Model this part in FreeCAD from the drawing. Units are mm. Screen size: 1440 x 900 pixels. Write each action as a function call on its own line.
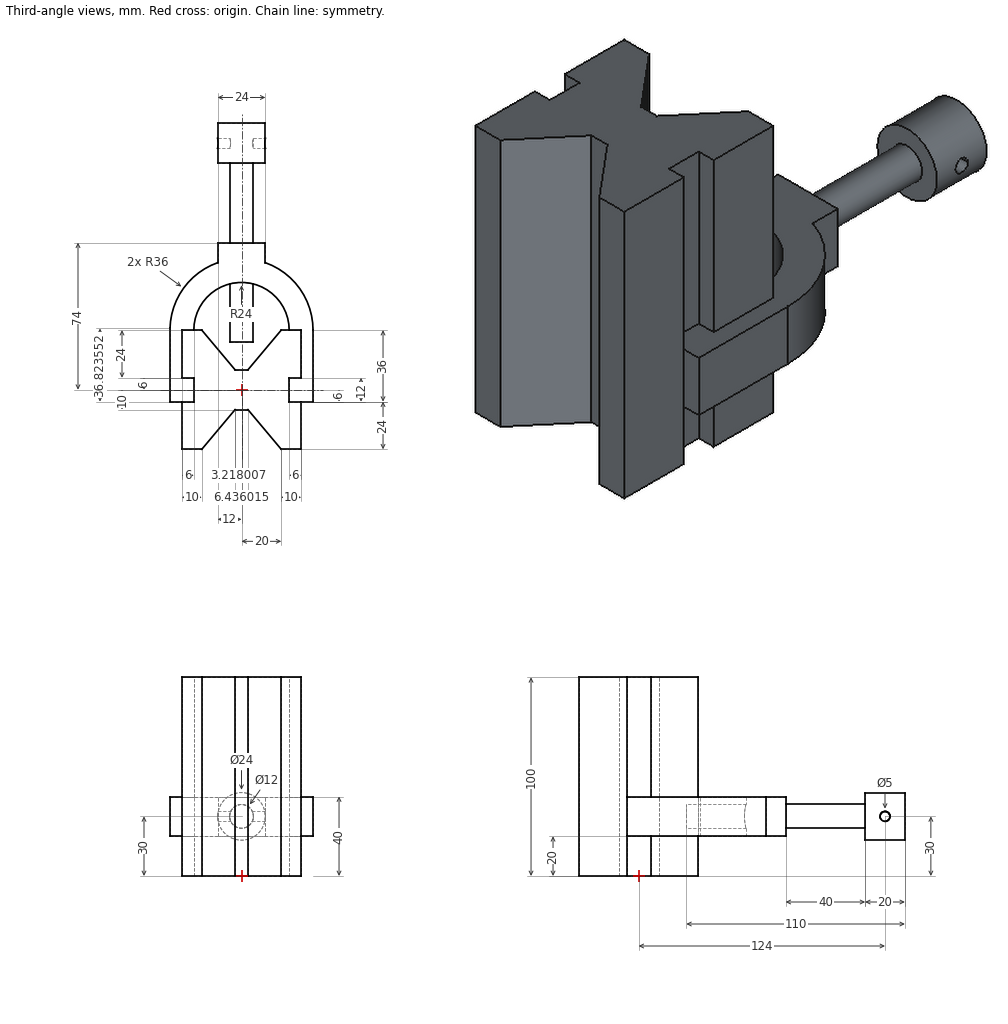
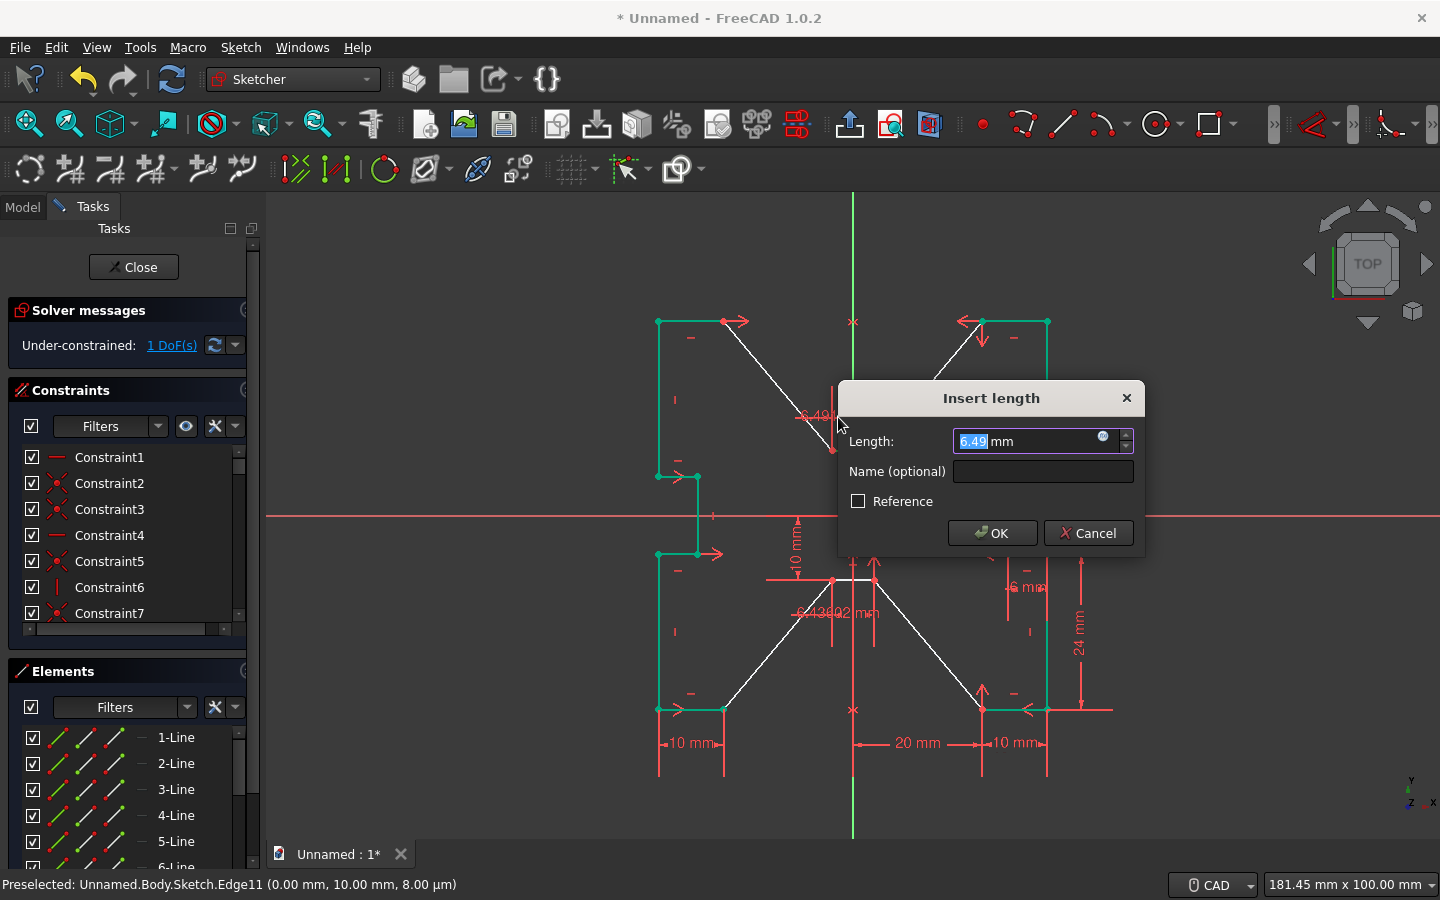
text(6.436015)
key(Return)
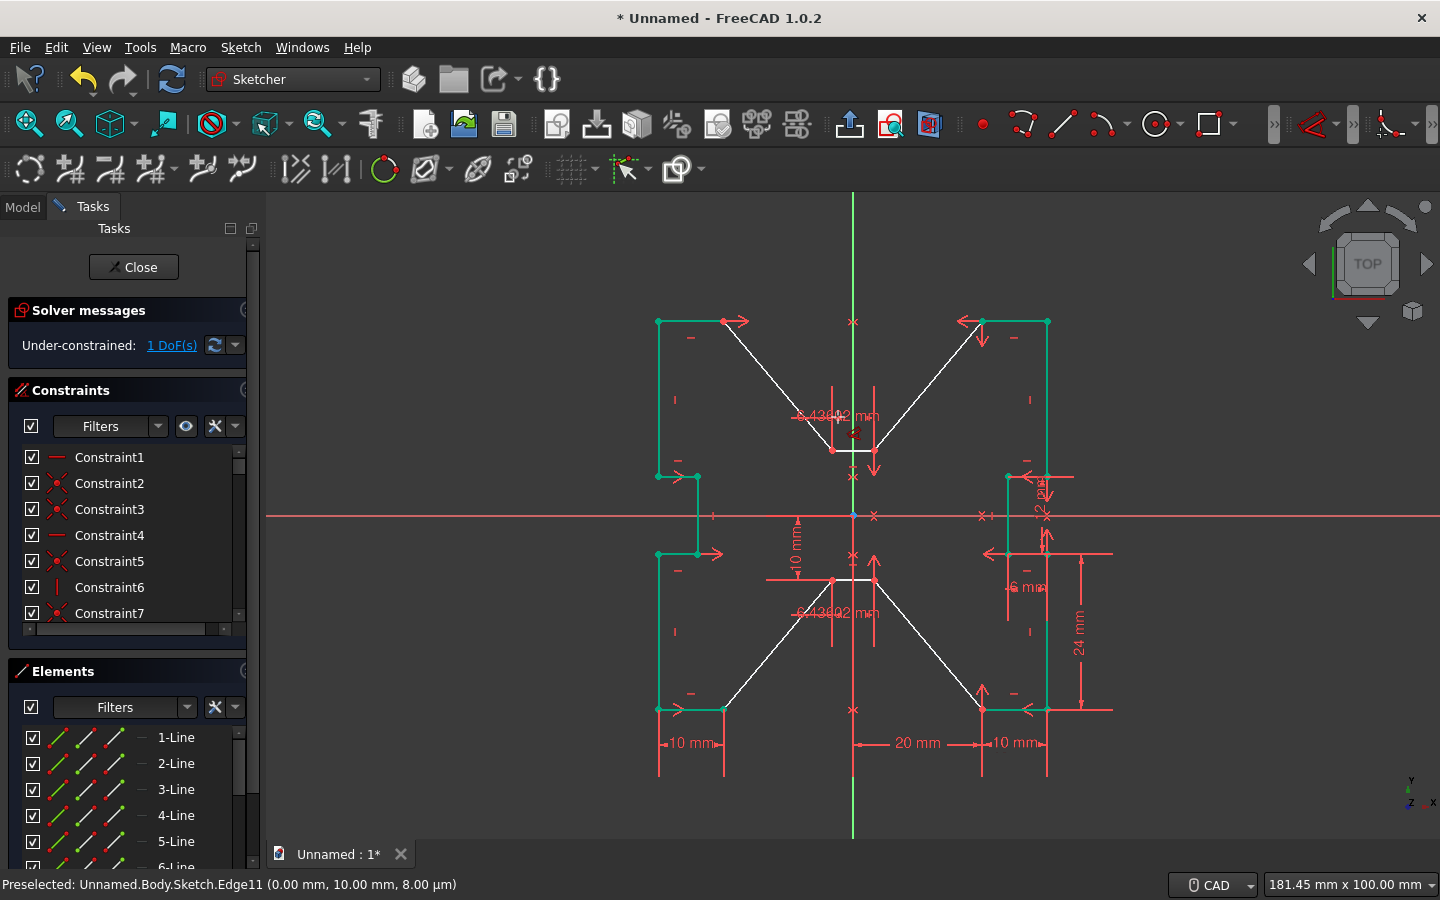
scroll(832, 580, up, 4)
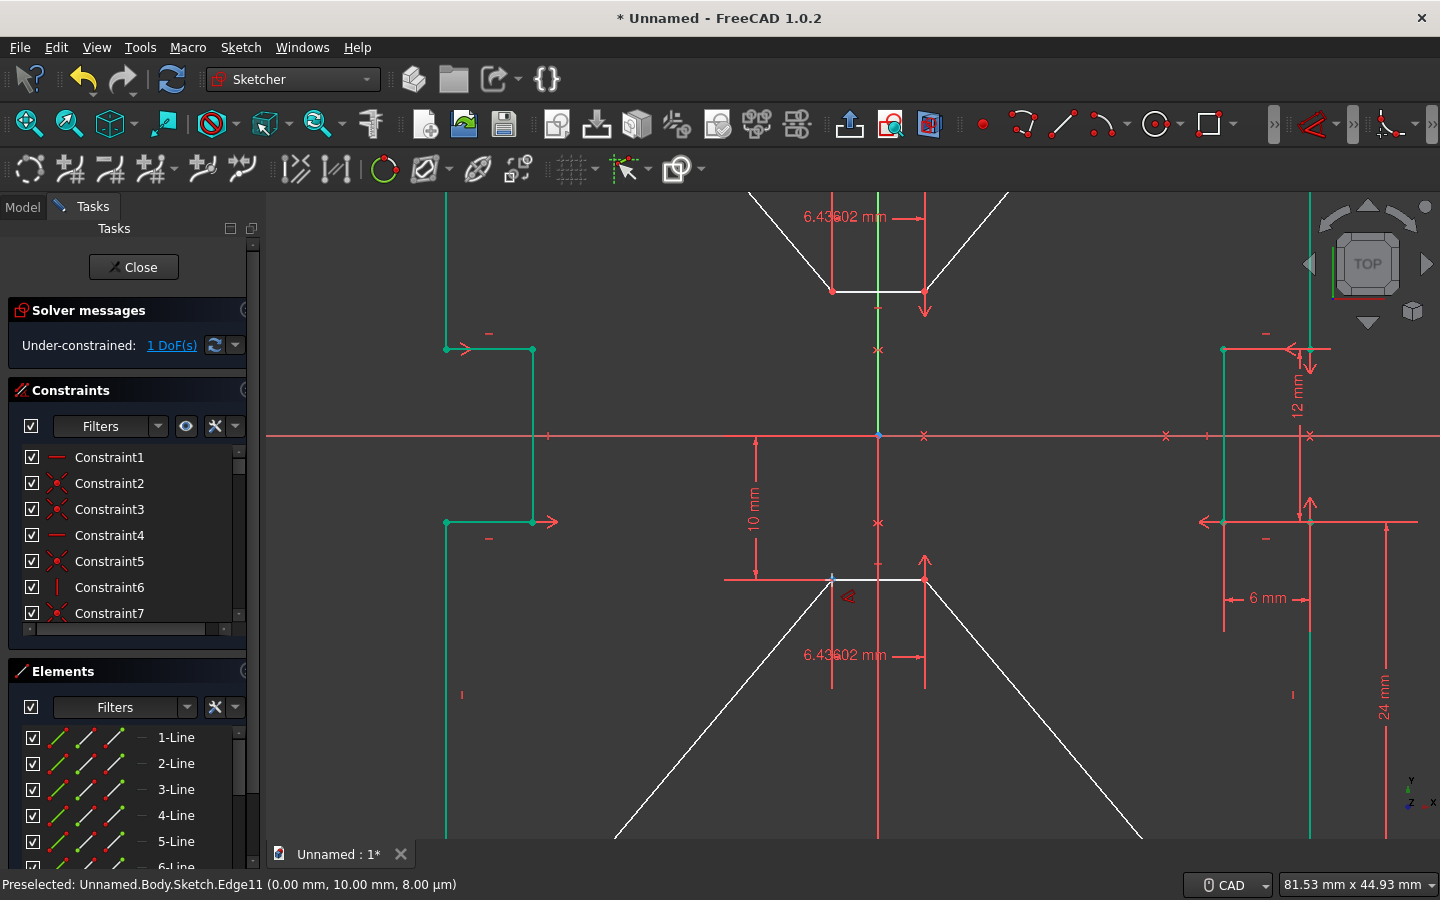
click(832, 580)
click(855, 614)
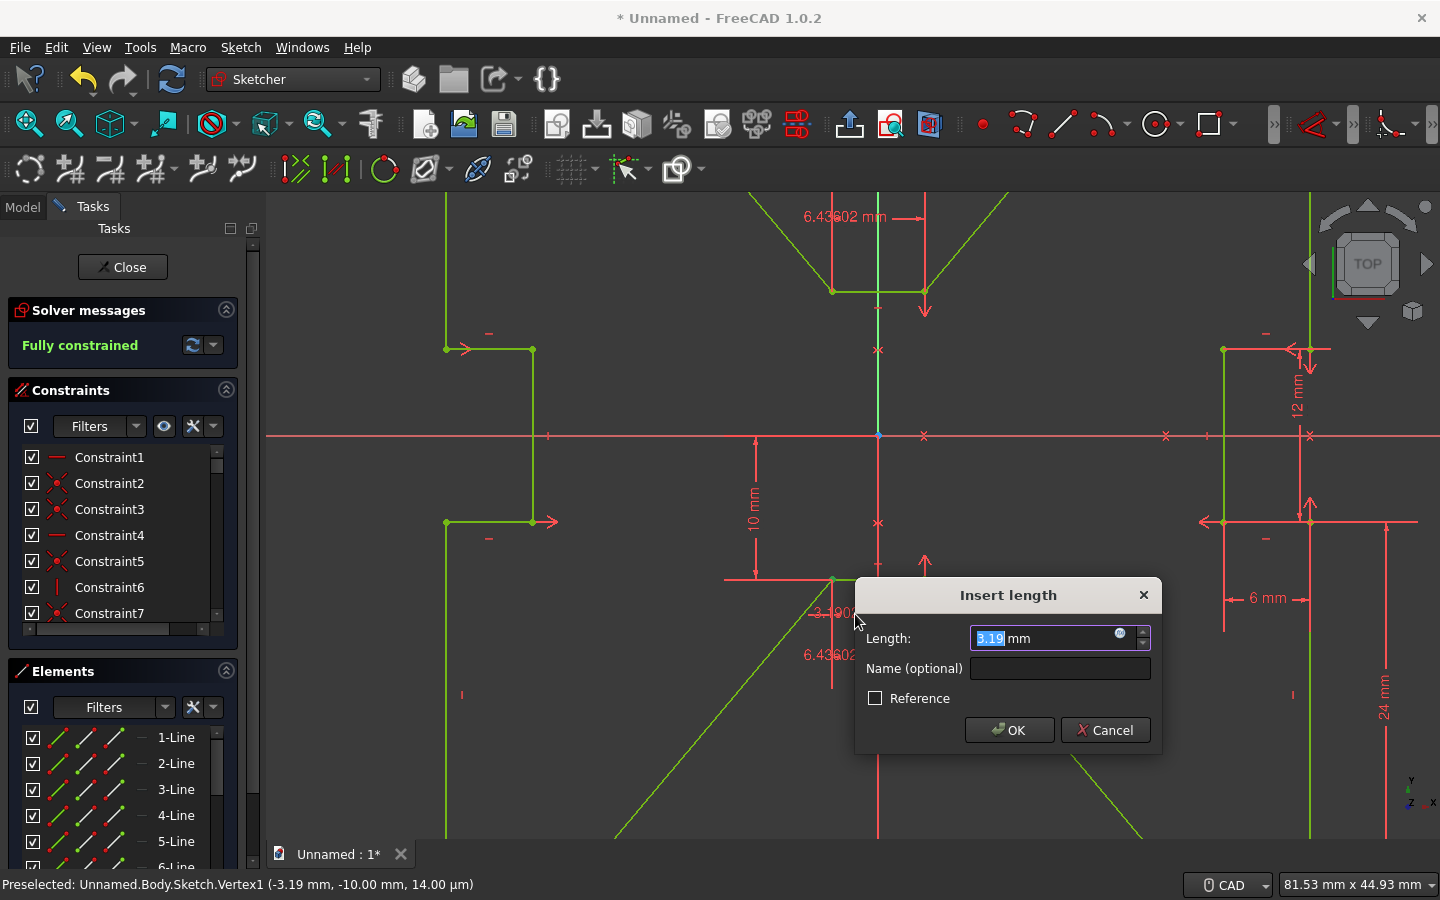
text(3.218007)
key(Return)
key(Escape)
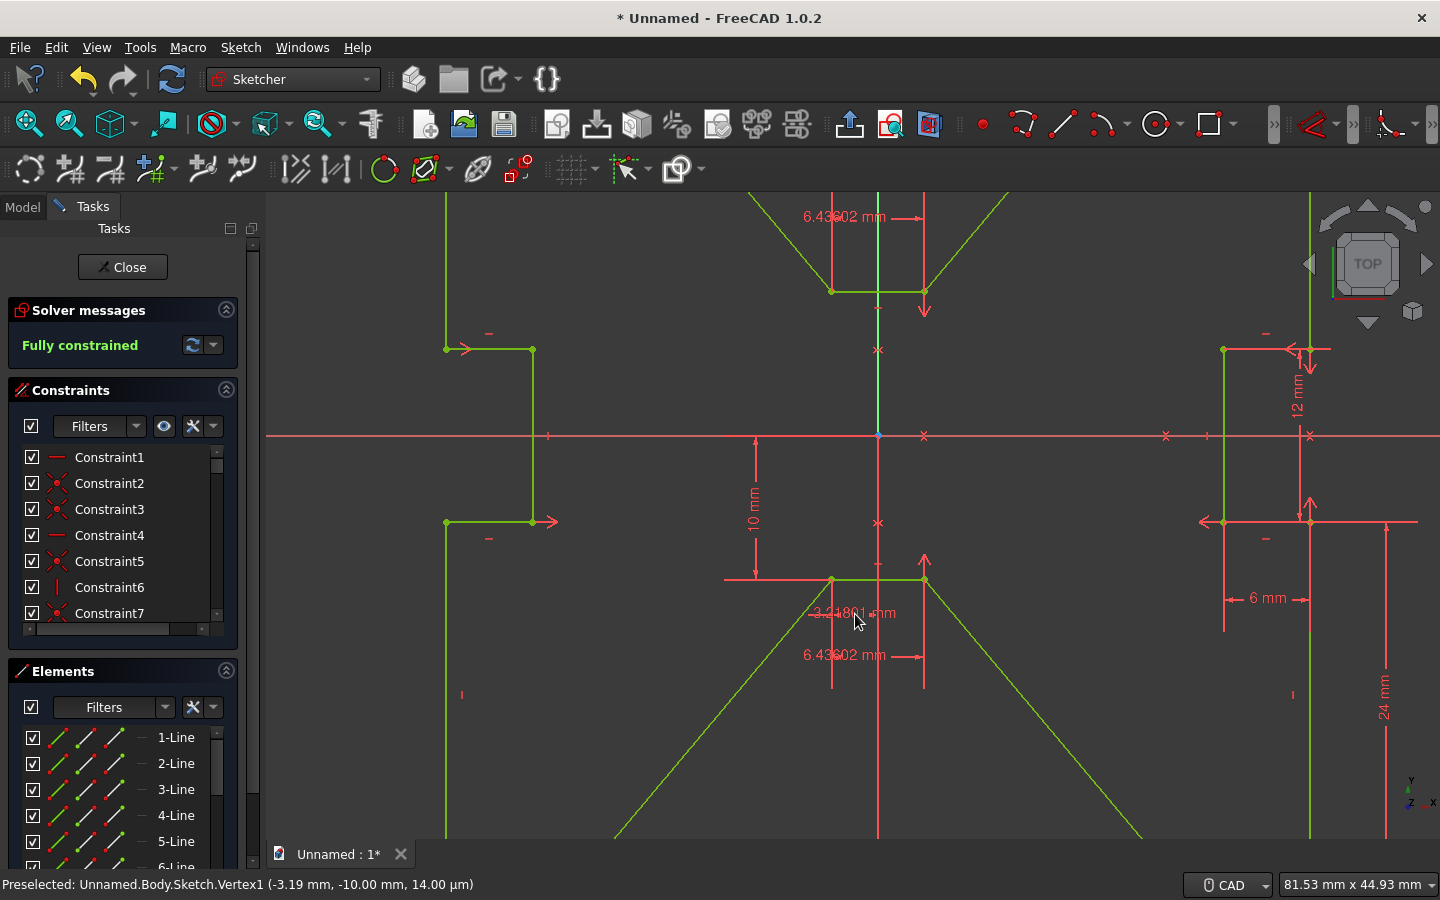
click(123, 267)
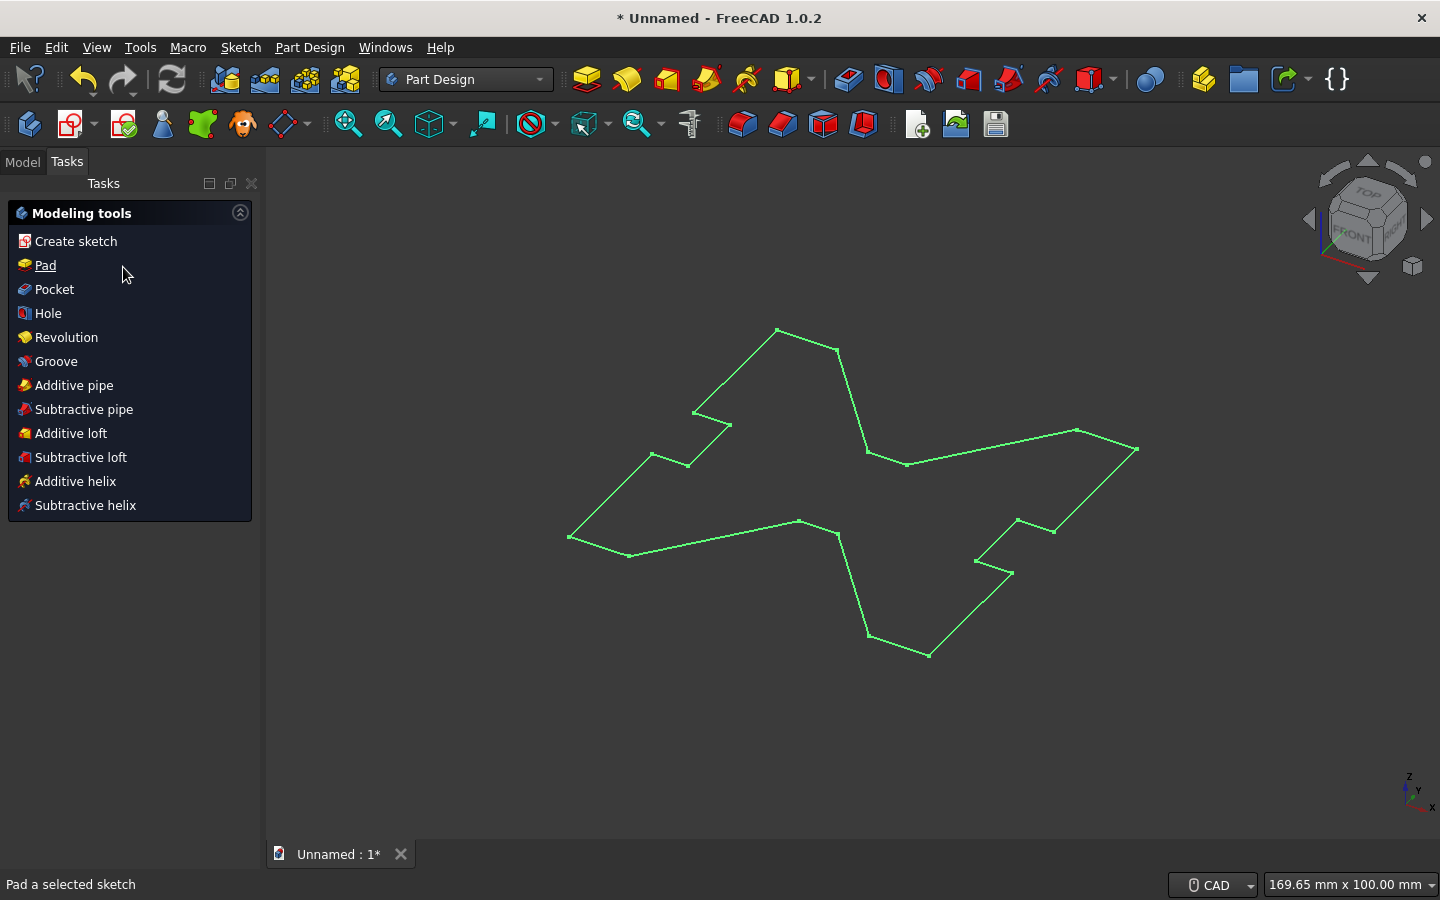
click(588, 80)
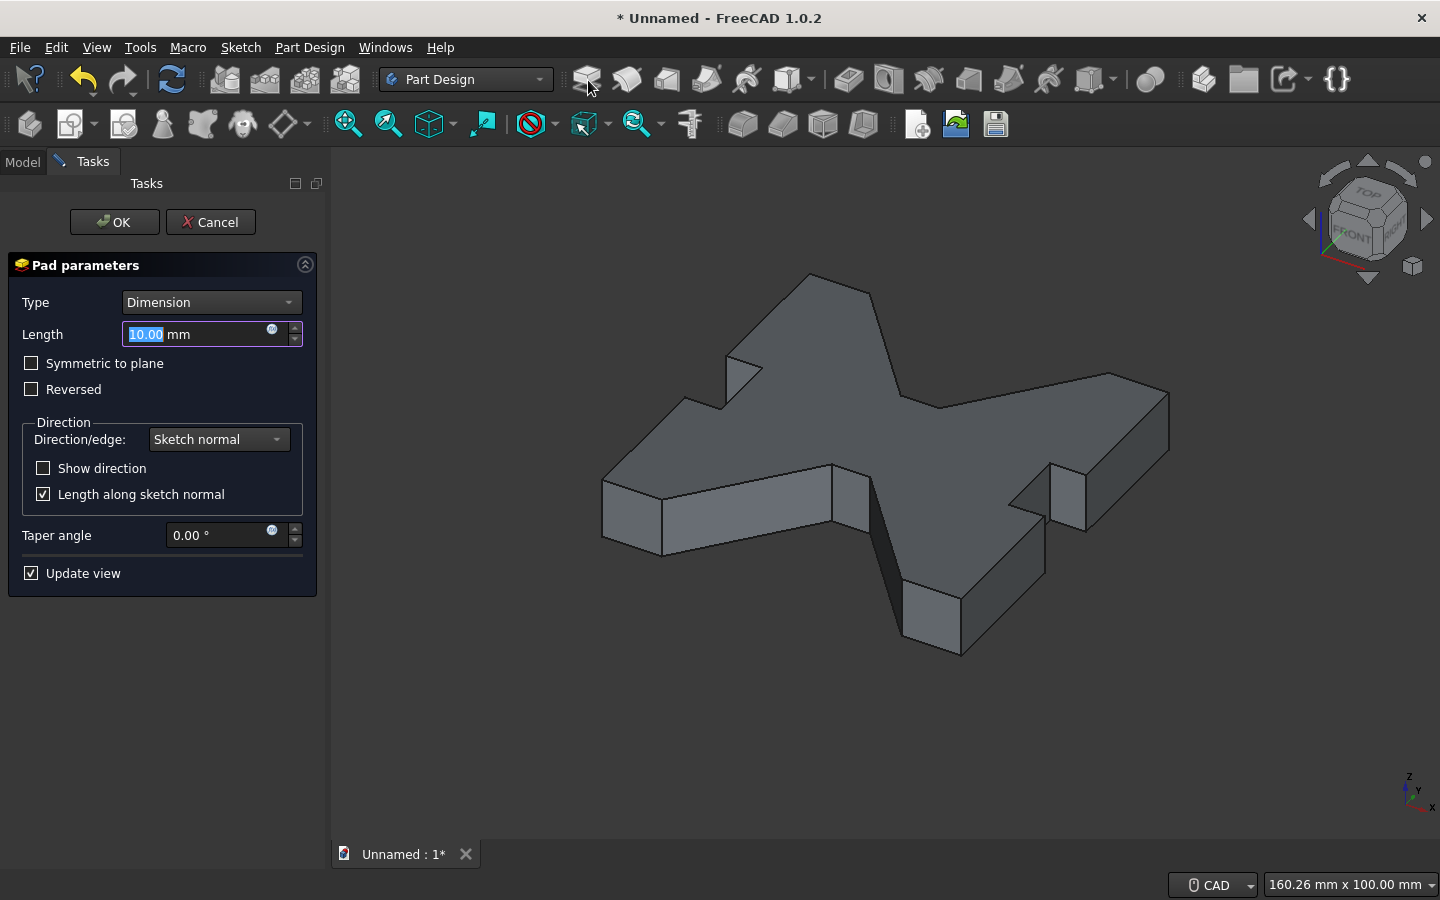
text(100)
key(Tab)